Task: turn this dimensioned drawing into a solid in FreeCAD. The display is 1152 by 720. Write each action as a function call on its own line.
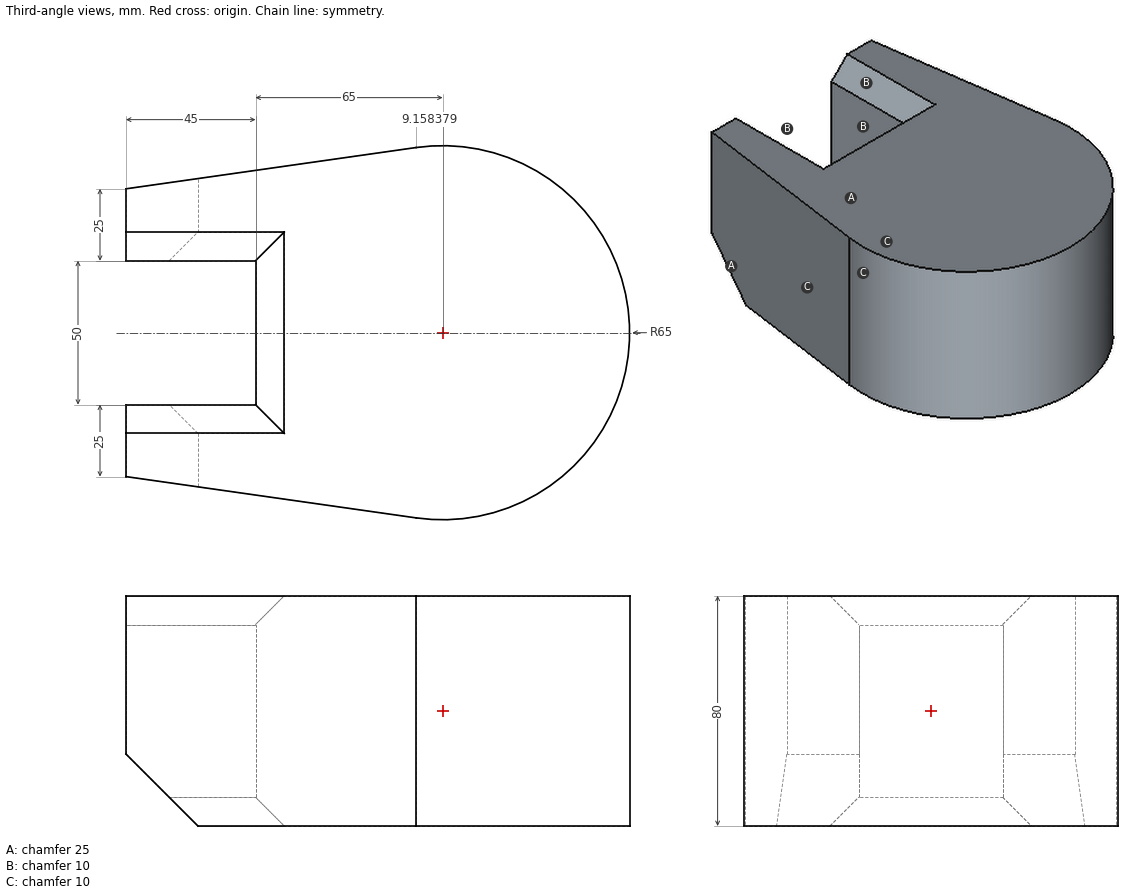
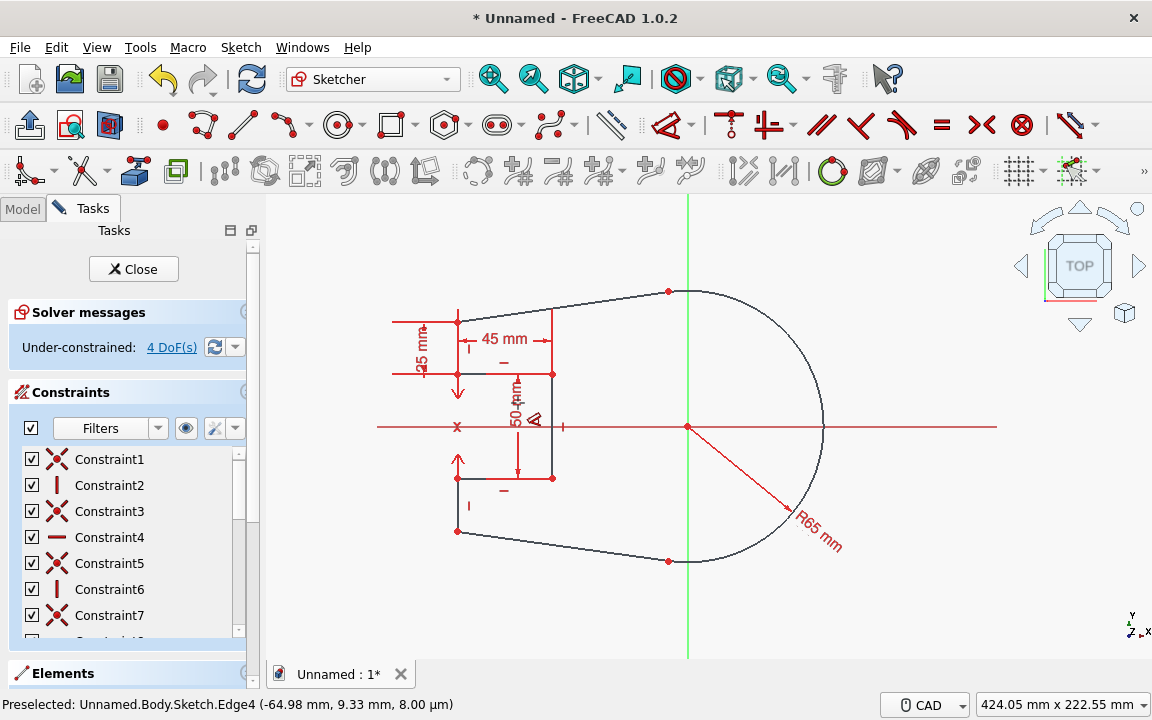
click(458, 495)
click(424, 505)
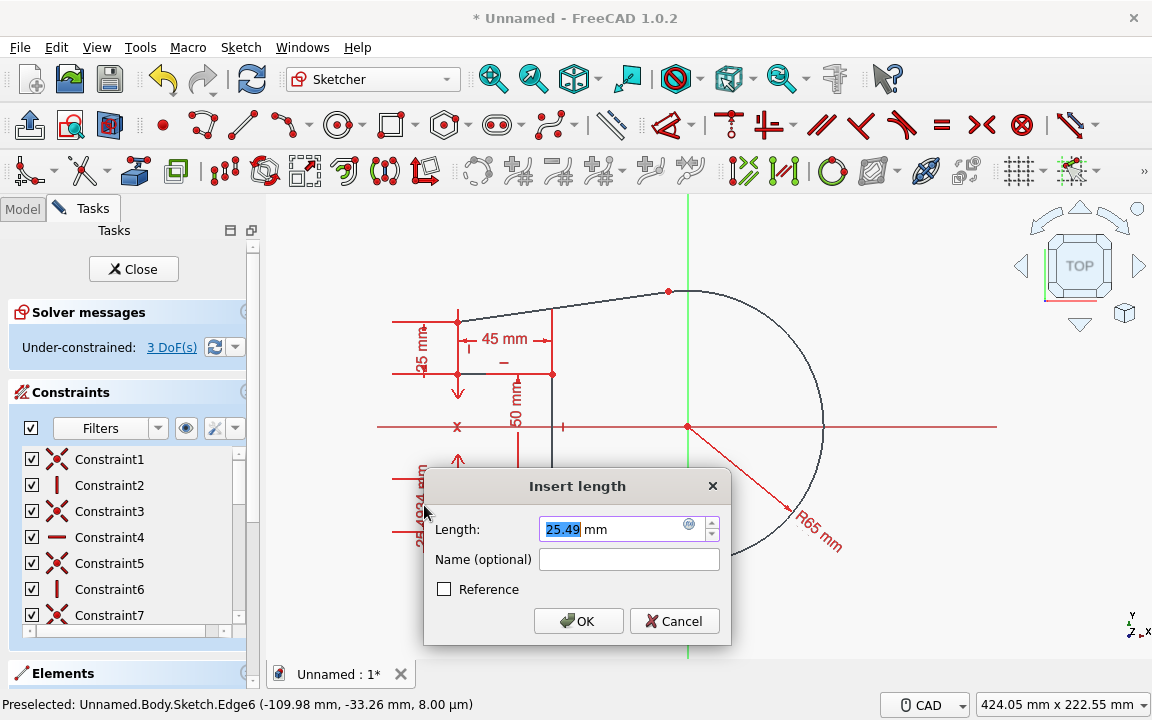
text(25)
key(Return)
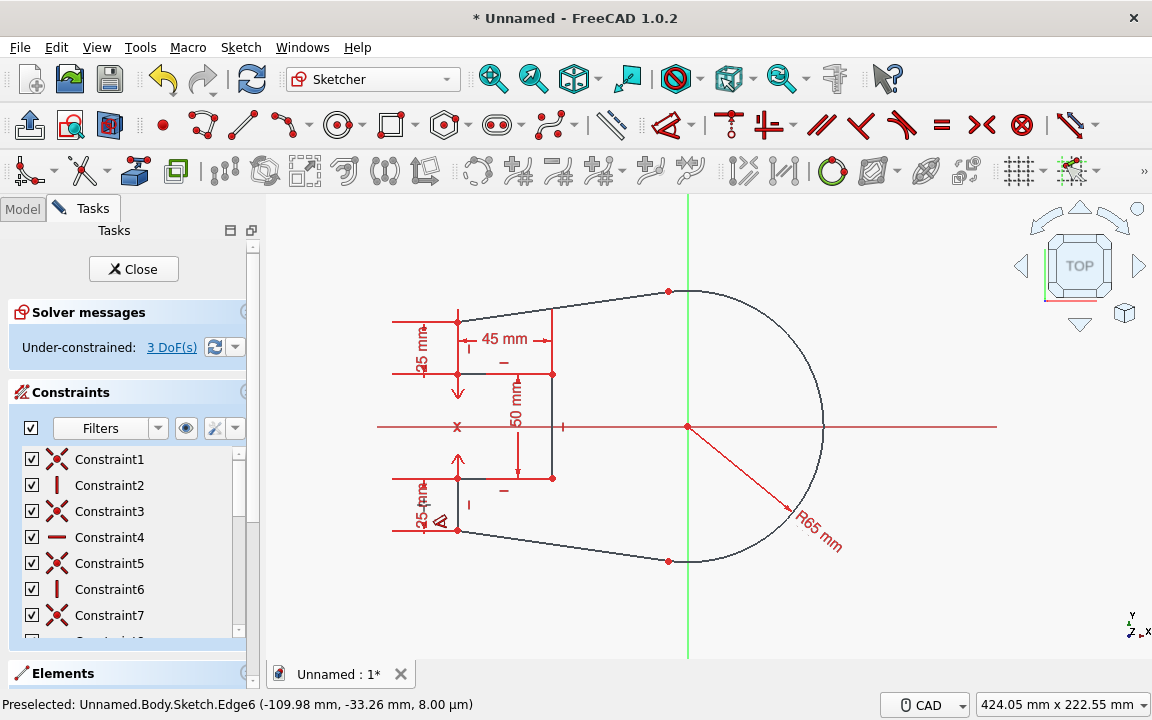
click(552, 374)
click(620, 340)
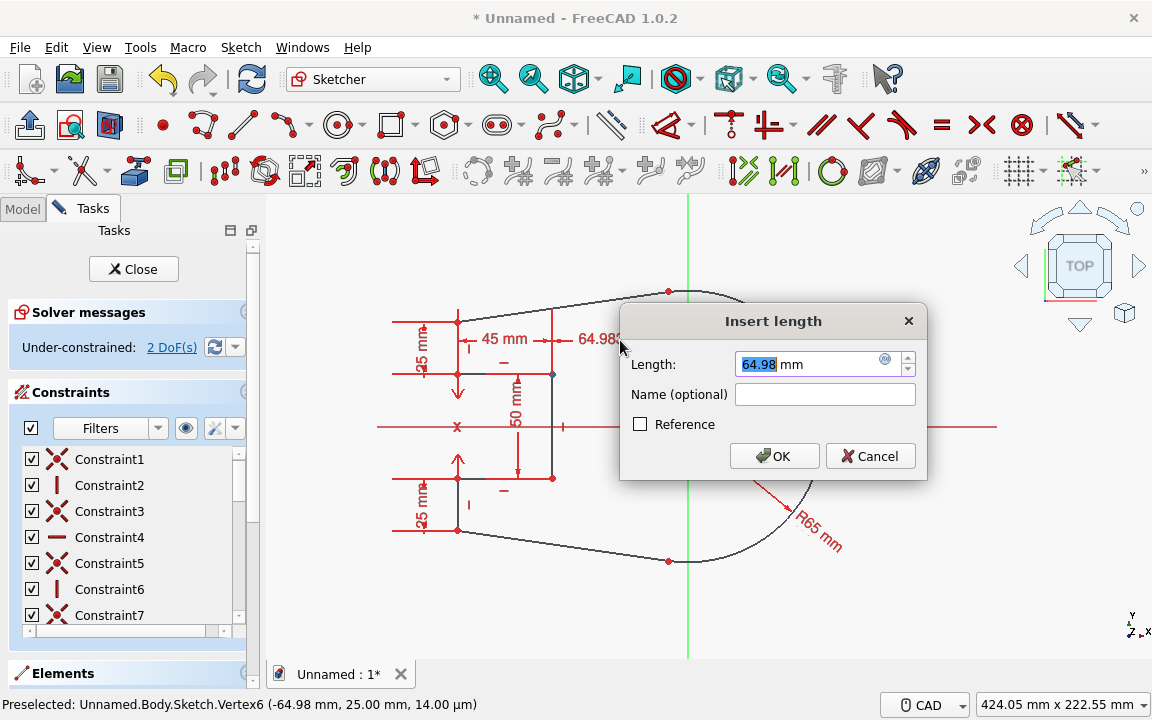
text(65)
key(Return)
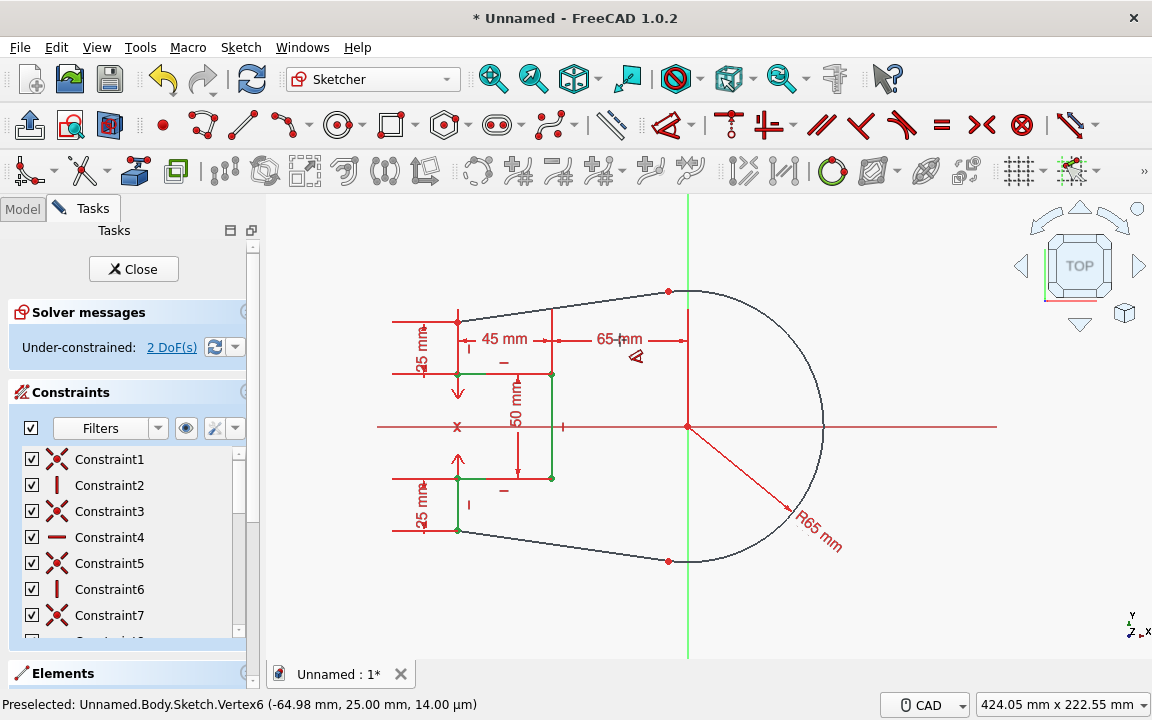
scroll(669, 292, up, 4)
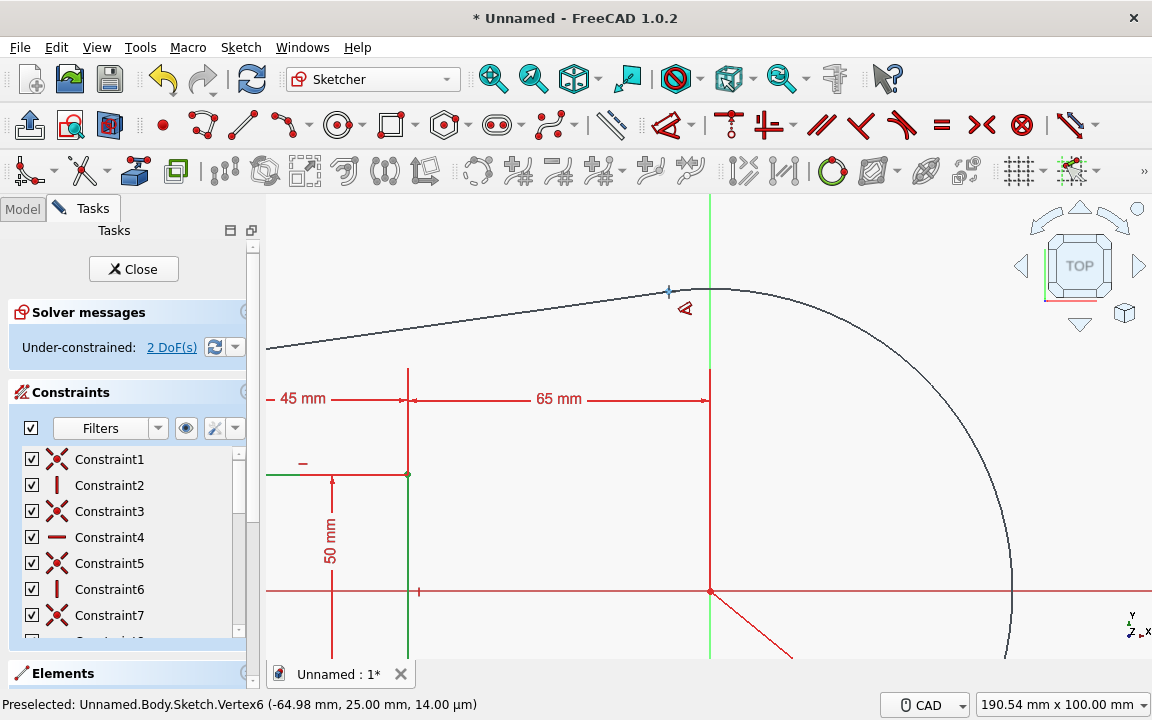
click(668, 292)
click(689, 258)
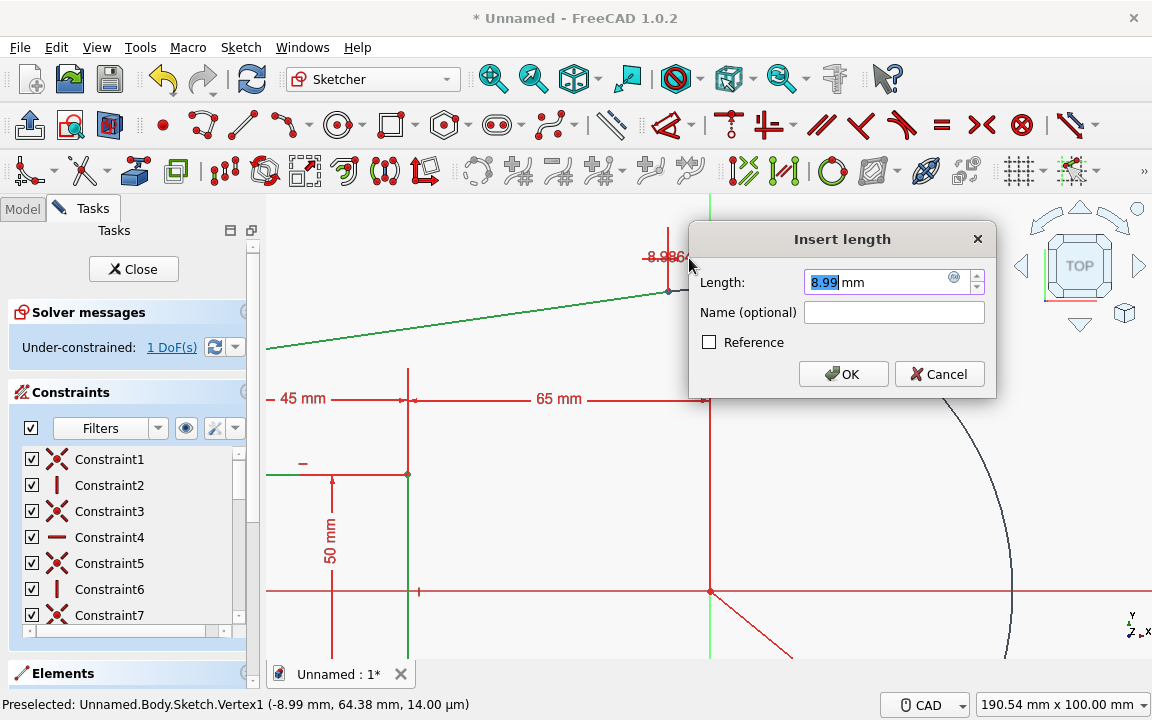
text(9.158379)
key(Return)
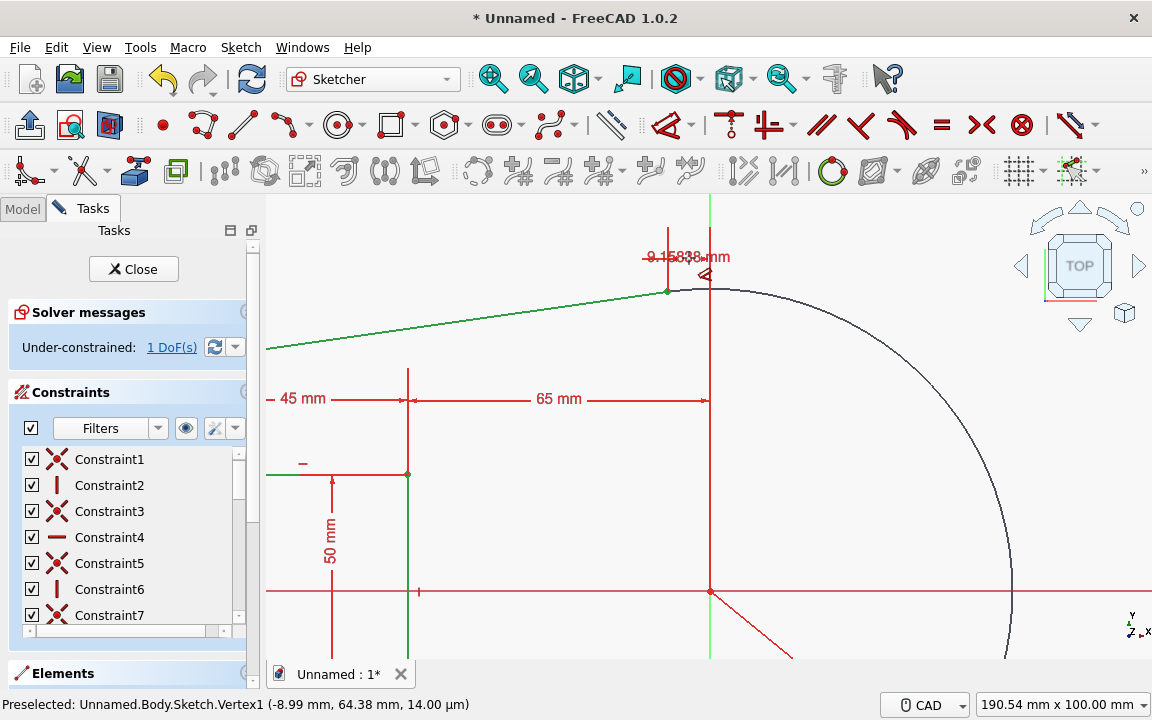
scroll(669, 292, down, 4)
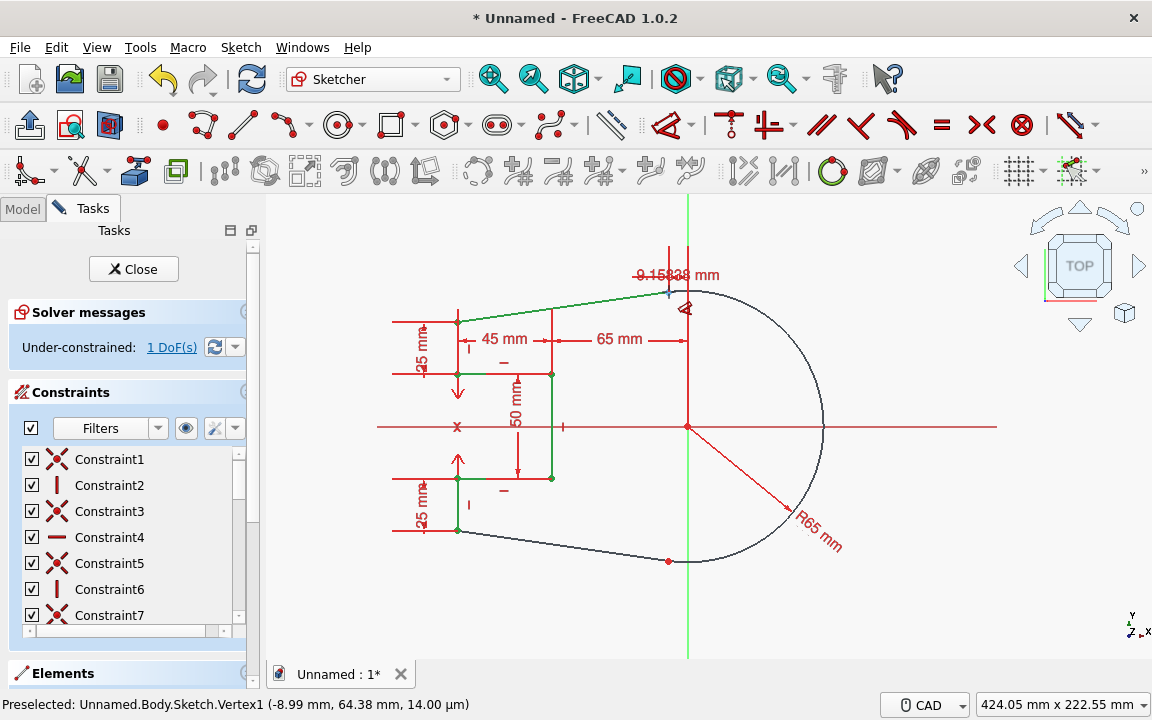
scroll(669, 561, up, 4)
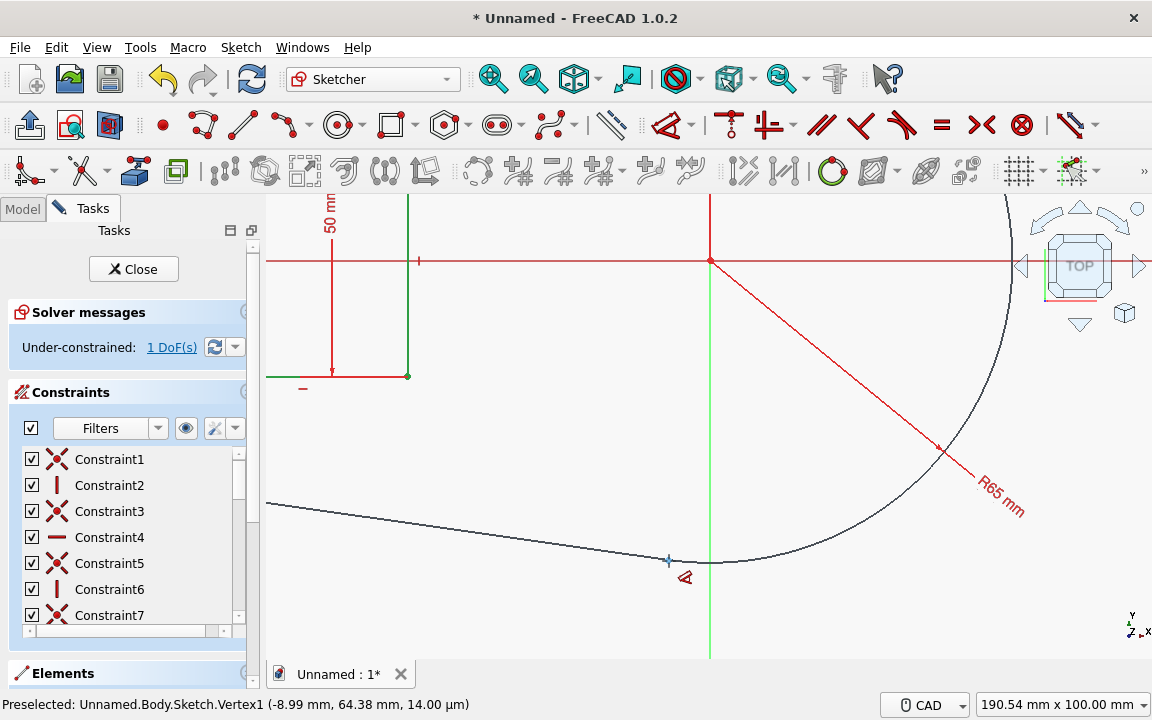
click(668, 560)
click(689, 594)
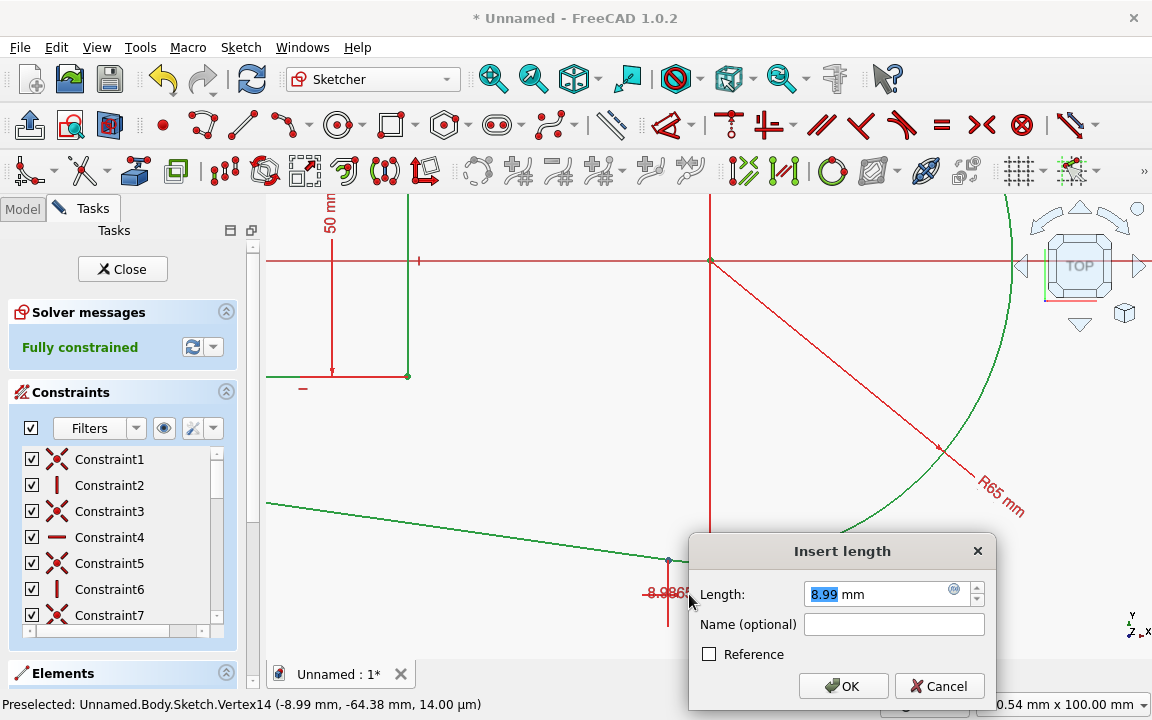
text(9.158379)
key(Return)
key(Escape)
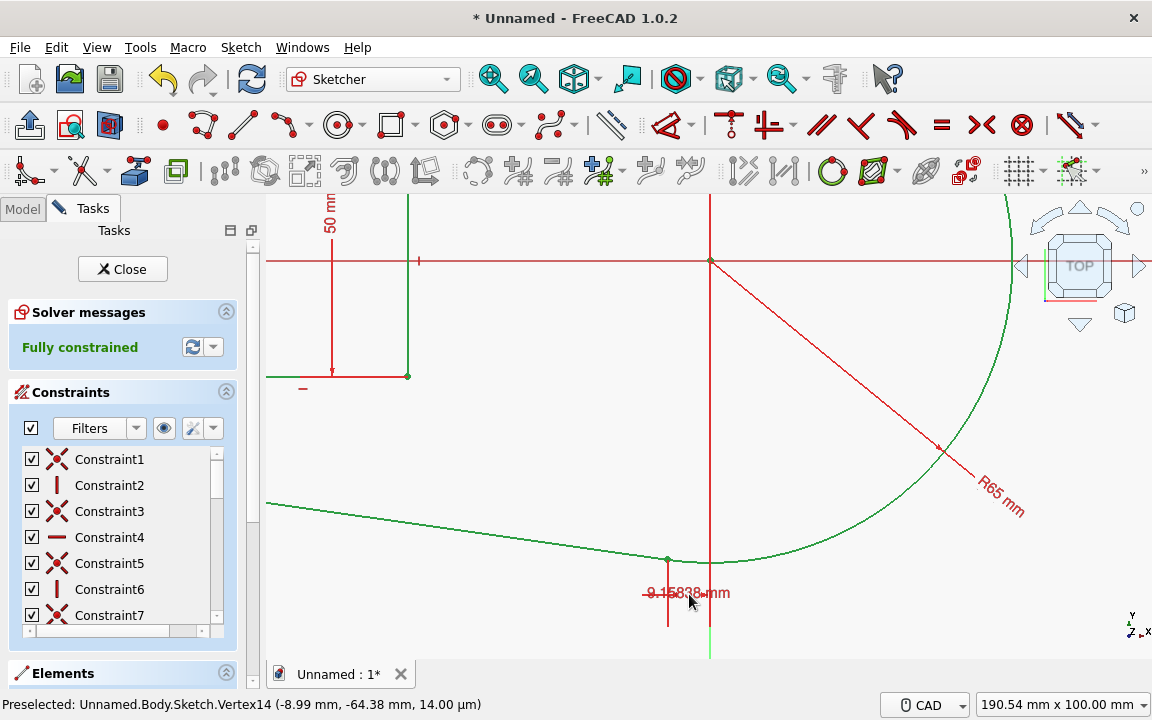
click(123, 269)